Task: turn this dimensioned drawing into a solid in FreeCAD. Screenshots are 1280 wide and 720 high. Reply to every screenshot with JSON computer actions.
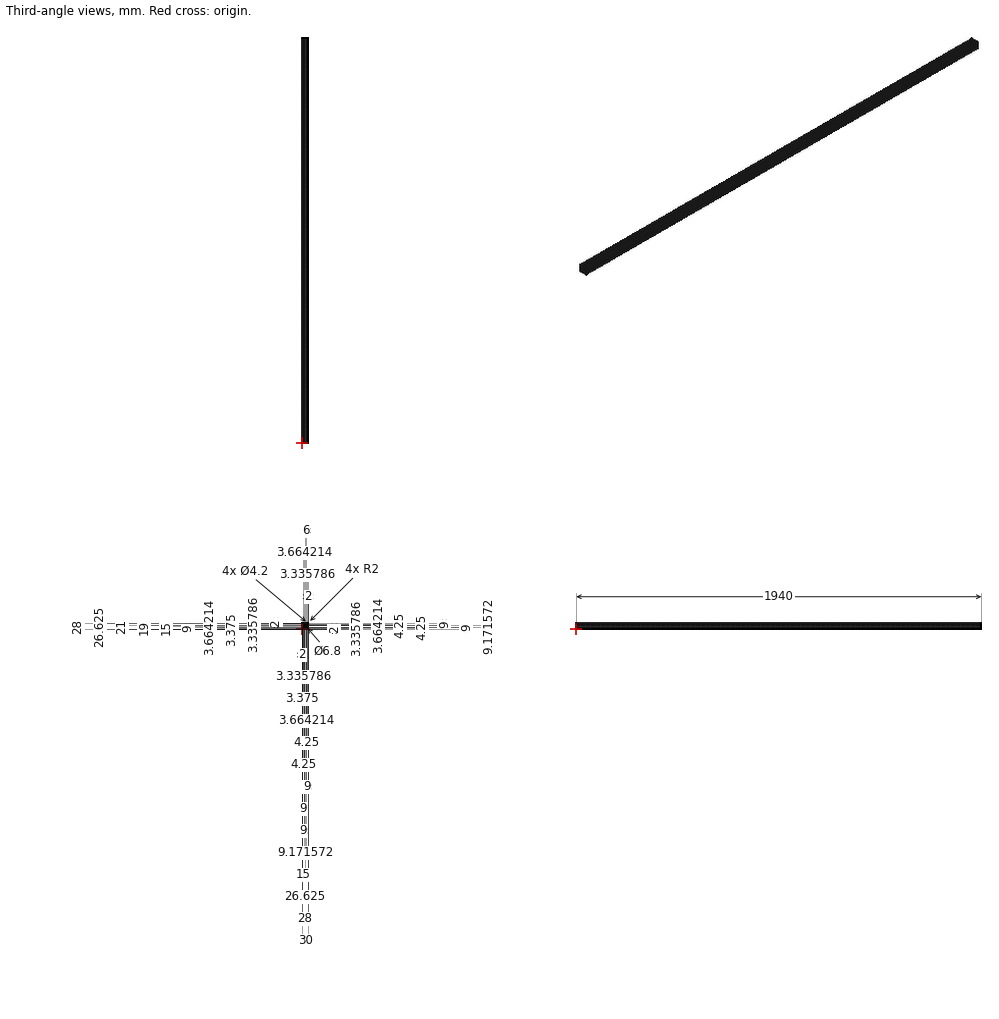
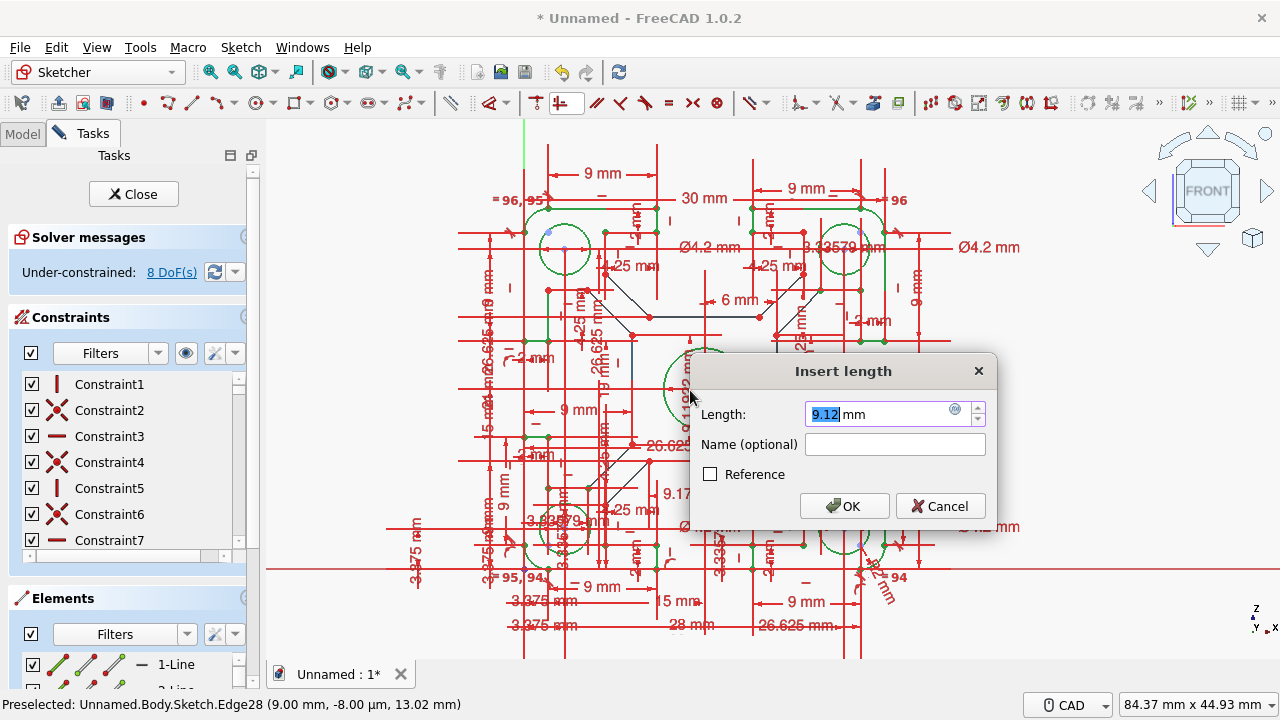
{"action": "type", "text": "9.171572"}
{"action": "key", "text": "Return"}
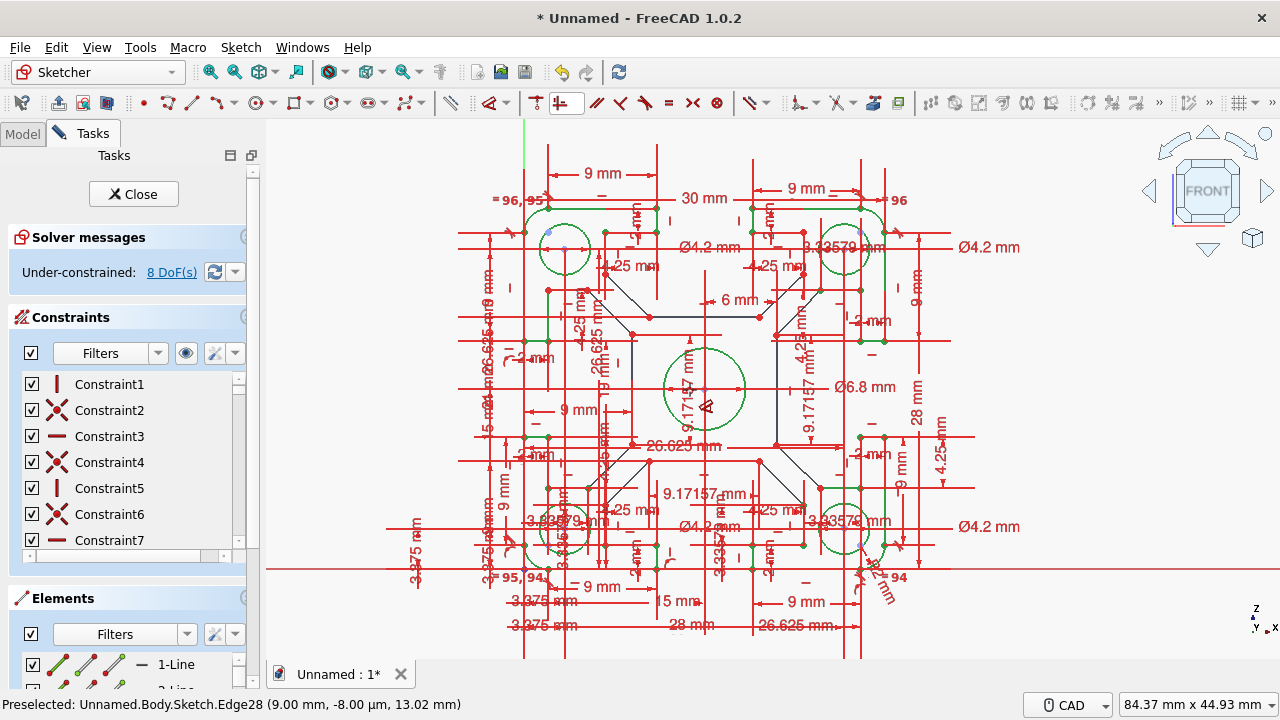
{"action": "left_click", "coordinate": [576, 290]}
{"action": "left_click", "coordinate": [559, 256]}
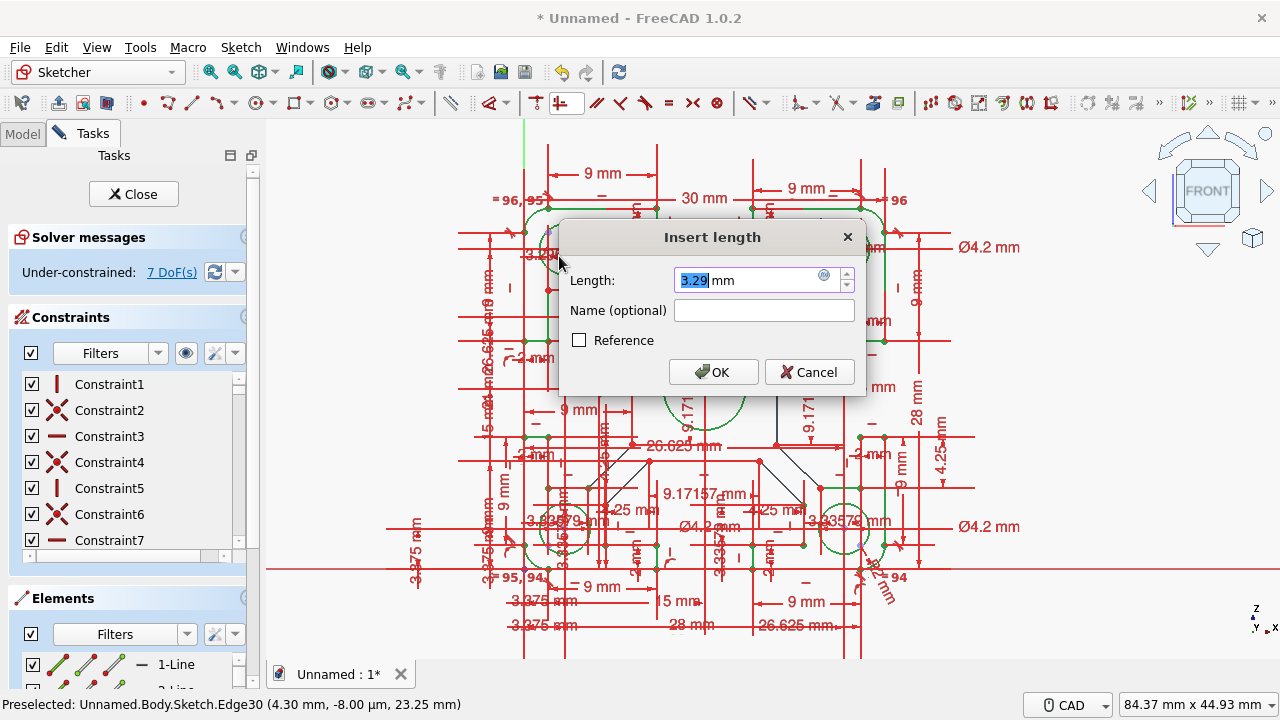
{"action": "type", "text": "3.335786"}
{"action": "key", "text": "Return"}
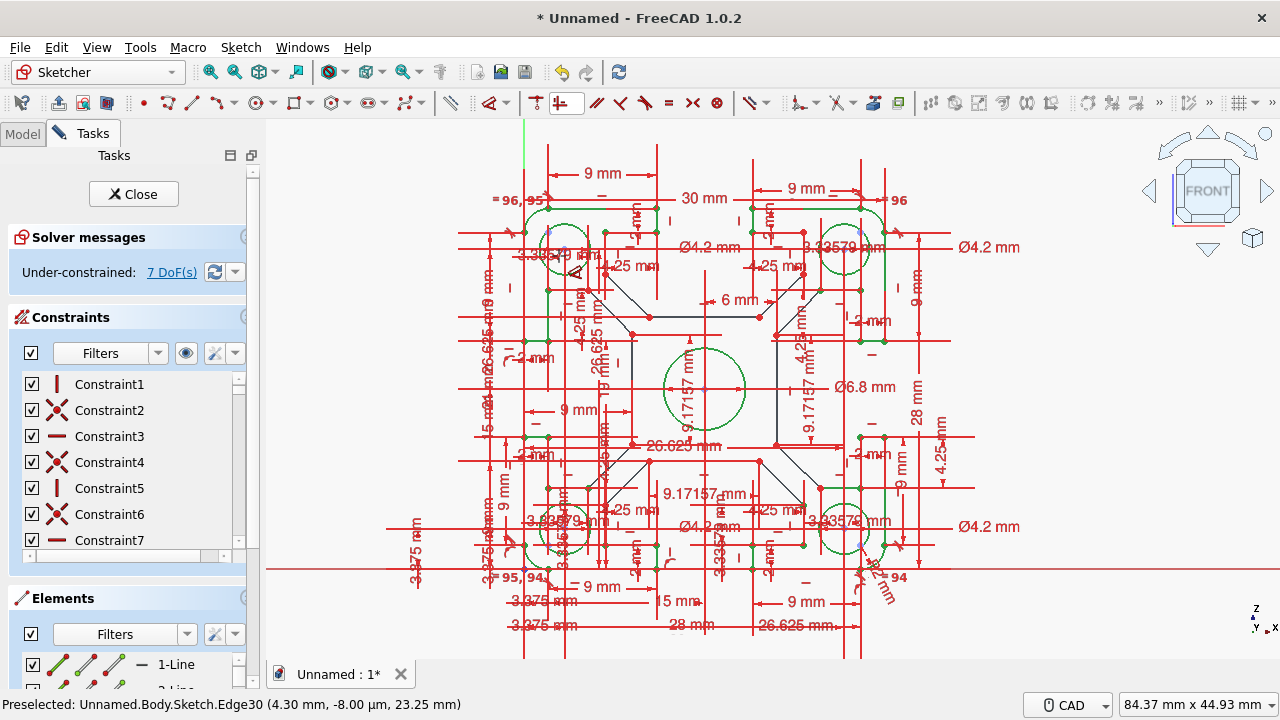
{"action": "left_click", "coordinate": [605, 245]}
{"action": "left_click", "coordinate": [663, 244]}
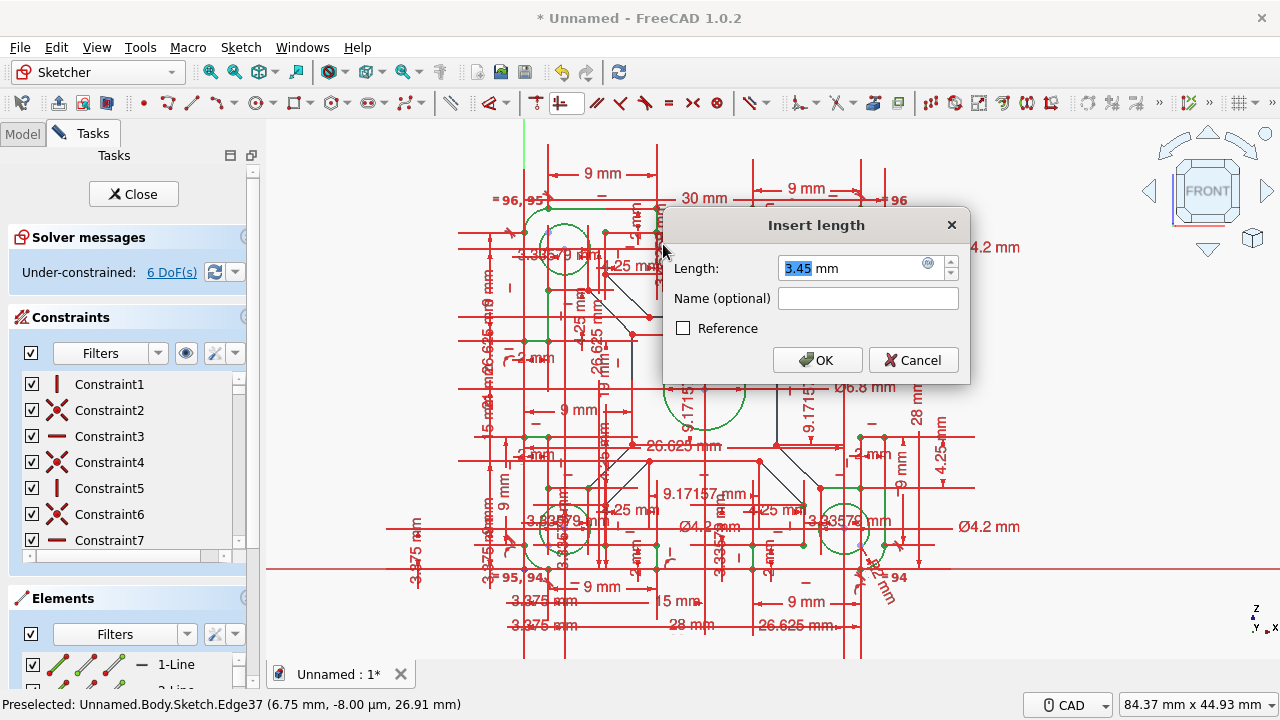
{"action": "type", "text": "3.335786"}
{"action": "key", "text": "Return"}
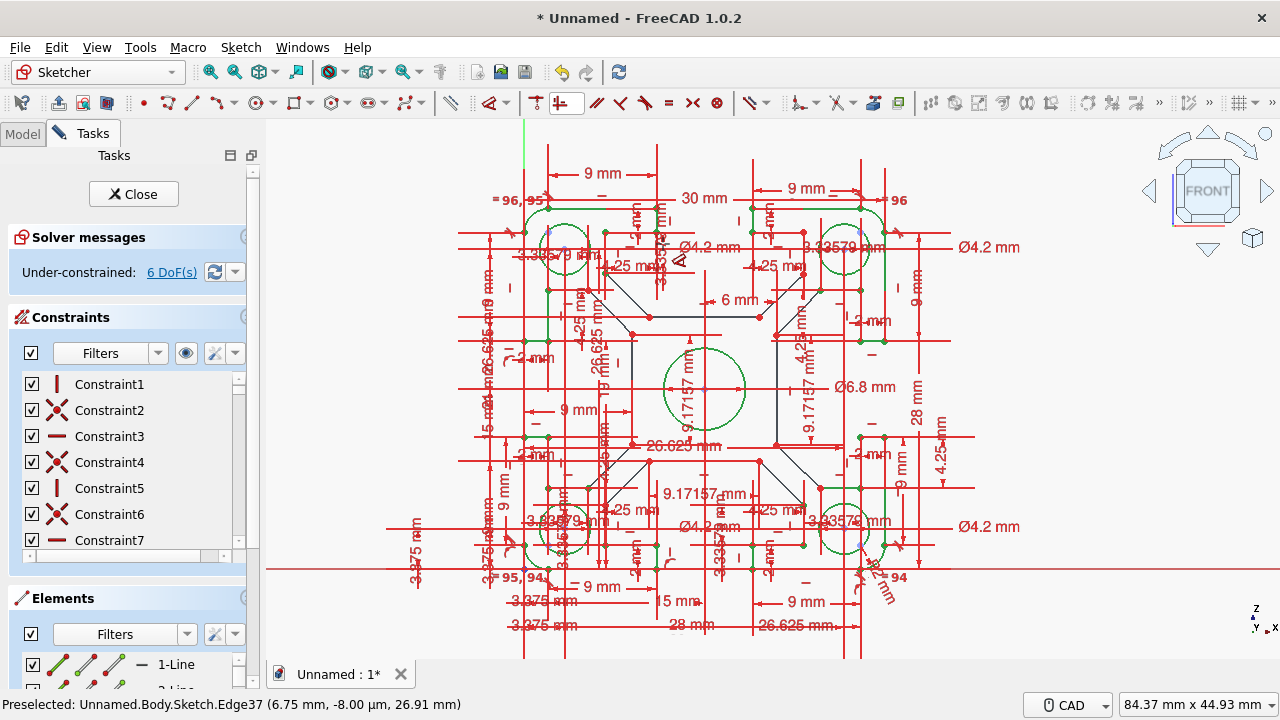
{"action": "left_click", "coordinate": [683, 317]}
{"action": "left_click", "coordinate": [705, 163]}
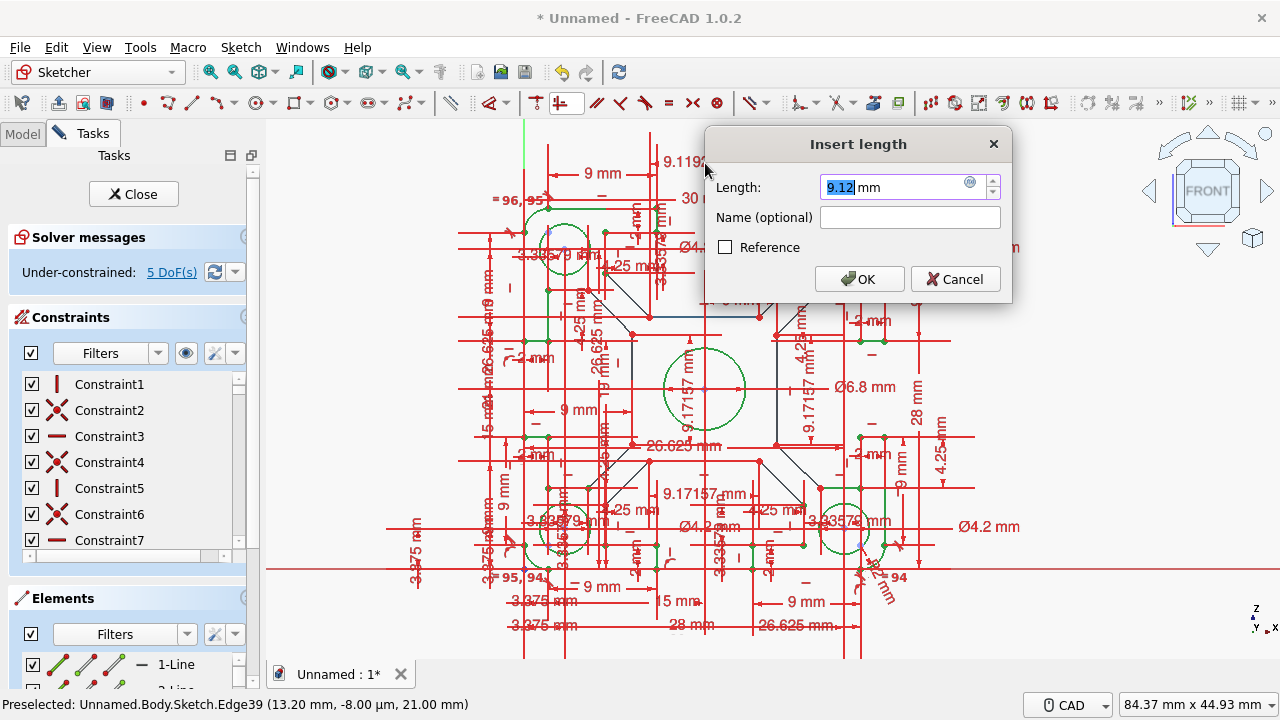
{"action": "type", "text": "9.171572"}
{"action": "key", "text": "Return"}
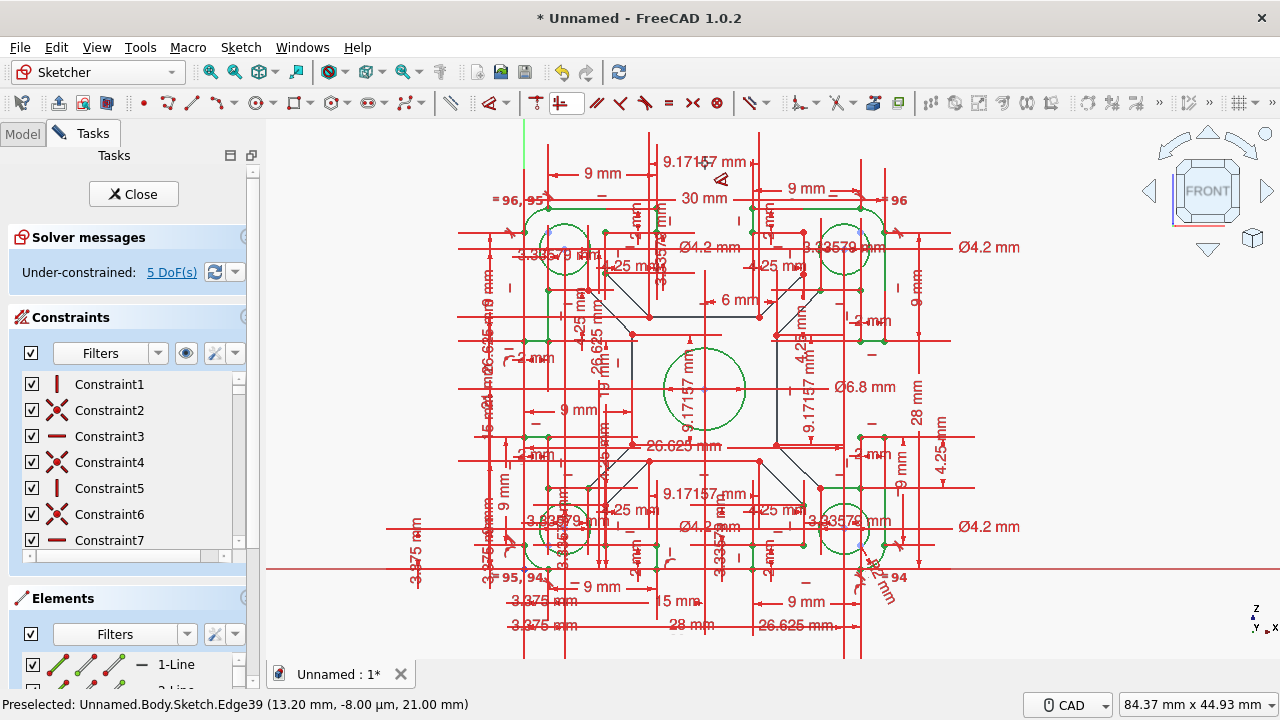
{"action": "left_click", "coordinate": [804, 262]}
{"action": "left_click", "coordinate": [746, 244]}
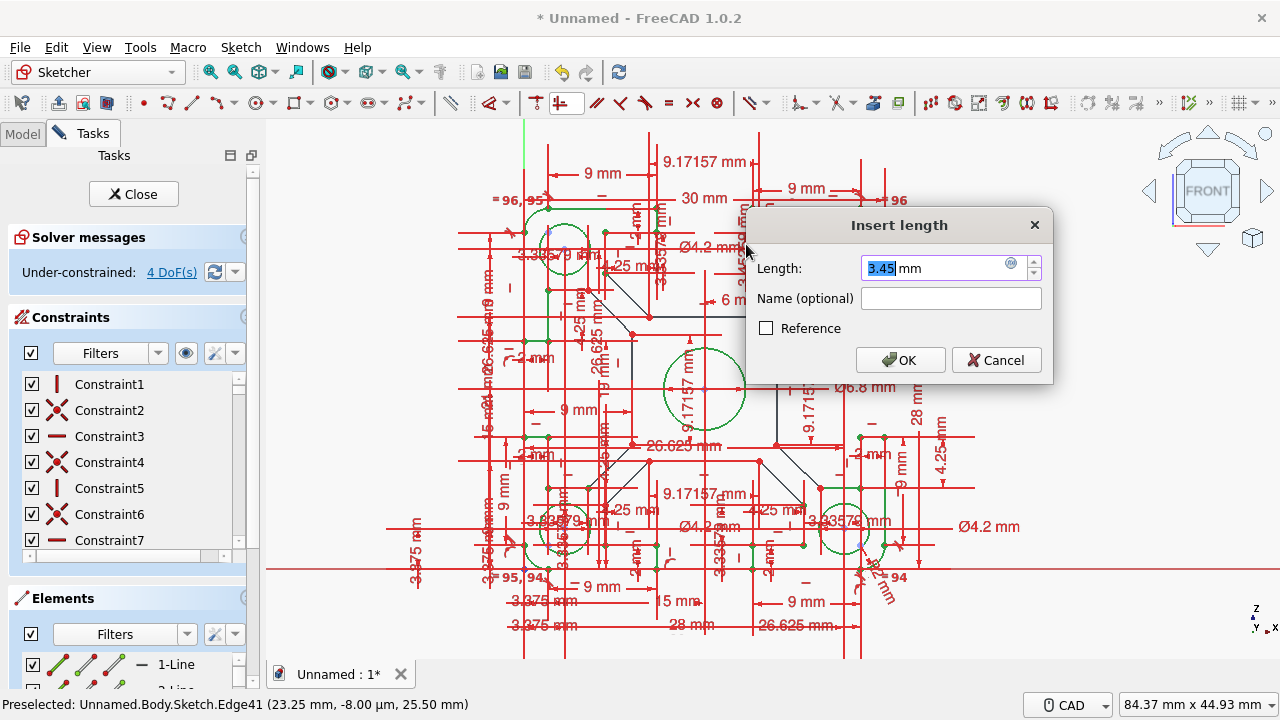
{"action": "type", "text": "3.335786"}
{"action": "key", "text": "Return"}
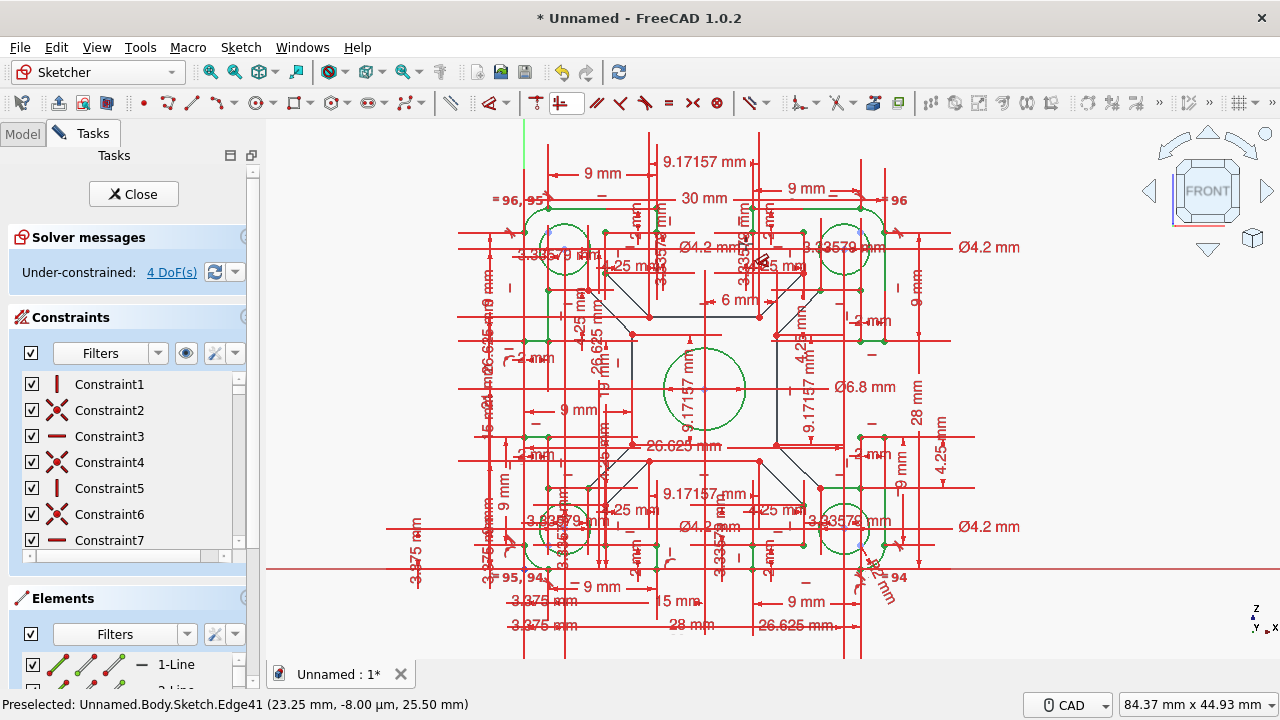
{"action": "left_click", "coordinate": [808, 304]}
{"action": "left_click", "coordinate": [951, 313]}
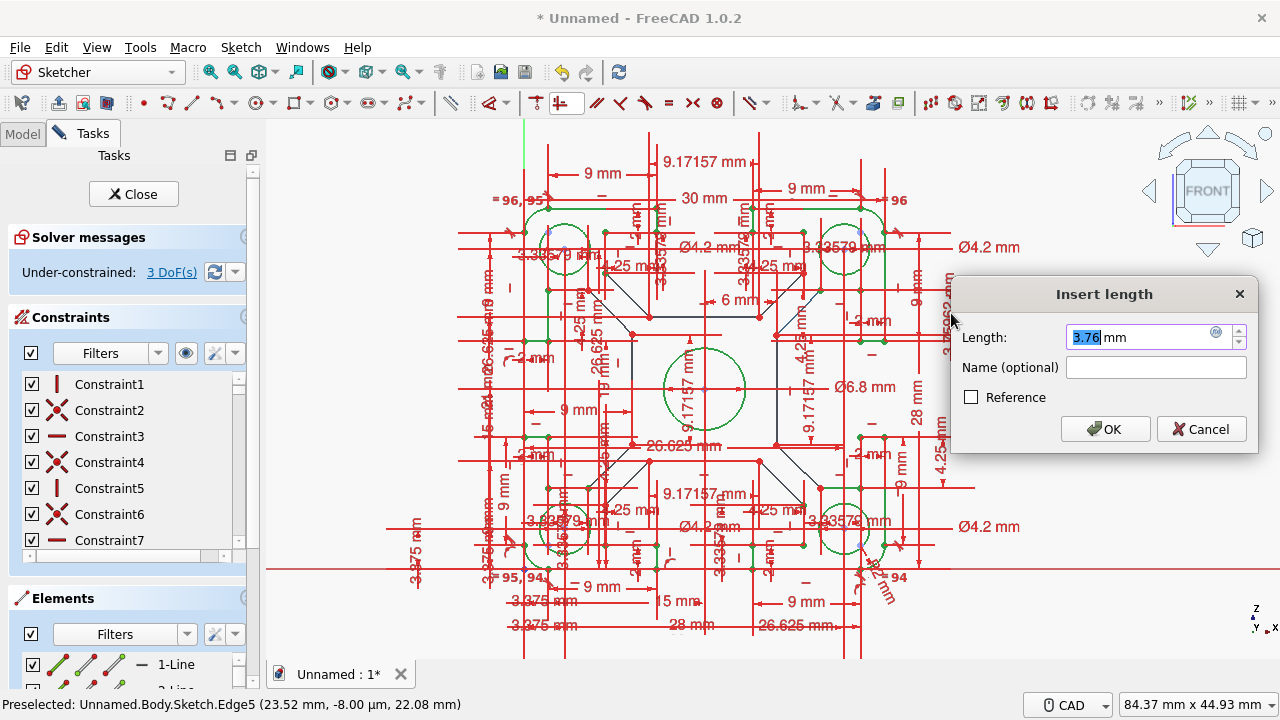
{"action": "type", "text": "3.664214"}
{"action": "key", "text": "Return"}